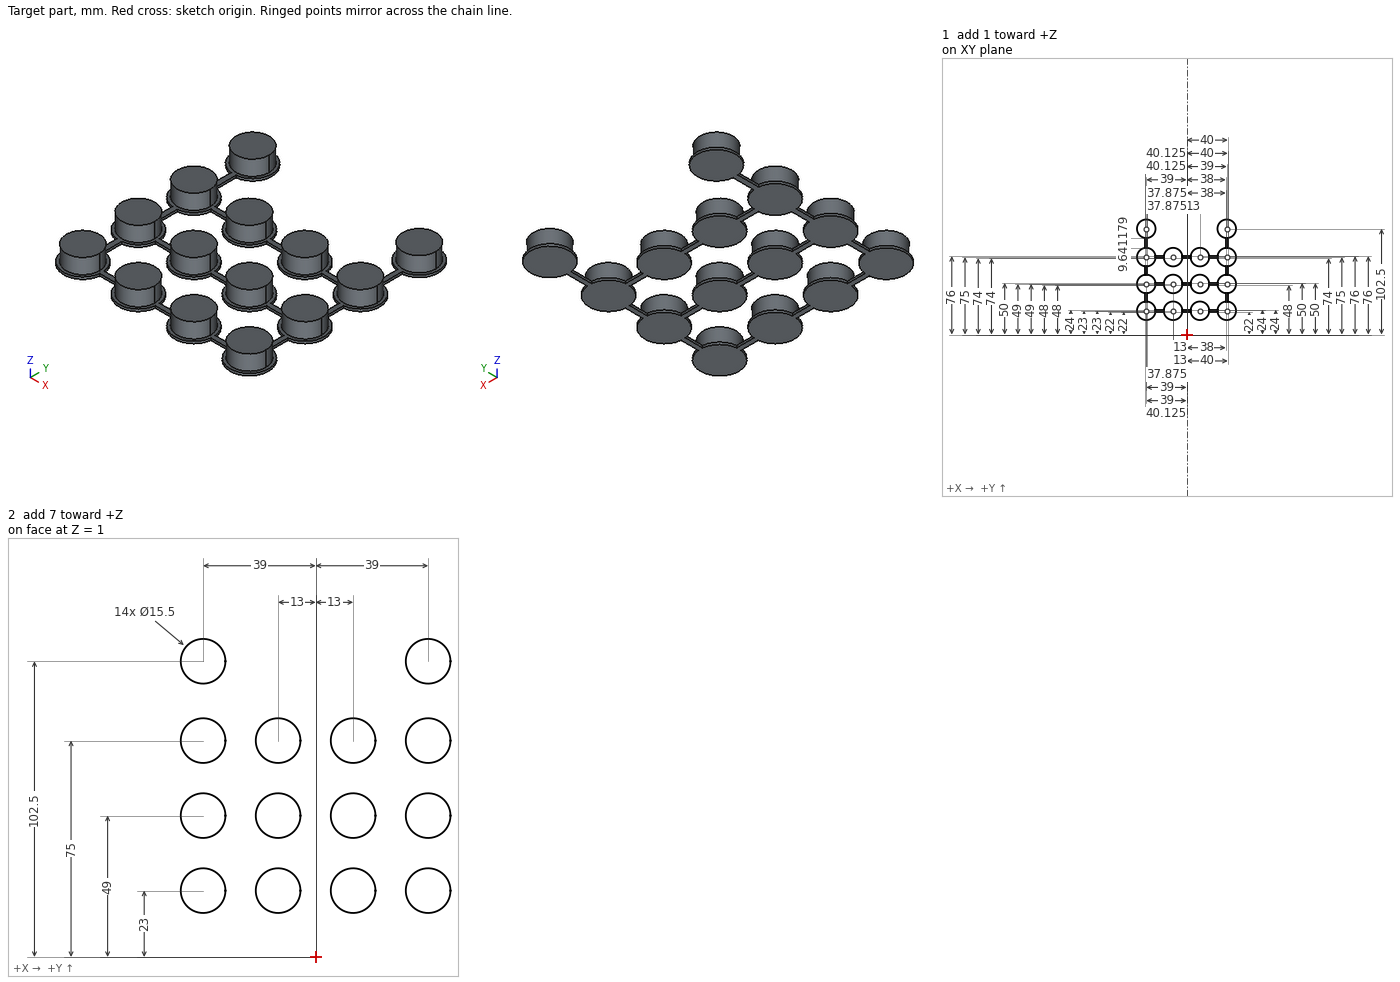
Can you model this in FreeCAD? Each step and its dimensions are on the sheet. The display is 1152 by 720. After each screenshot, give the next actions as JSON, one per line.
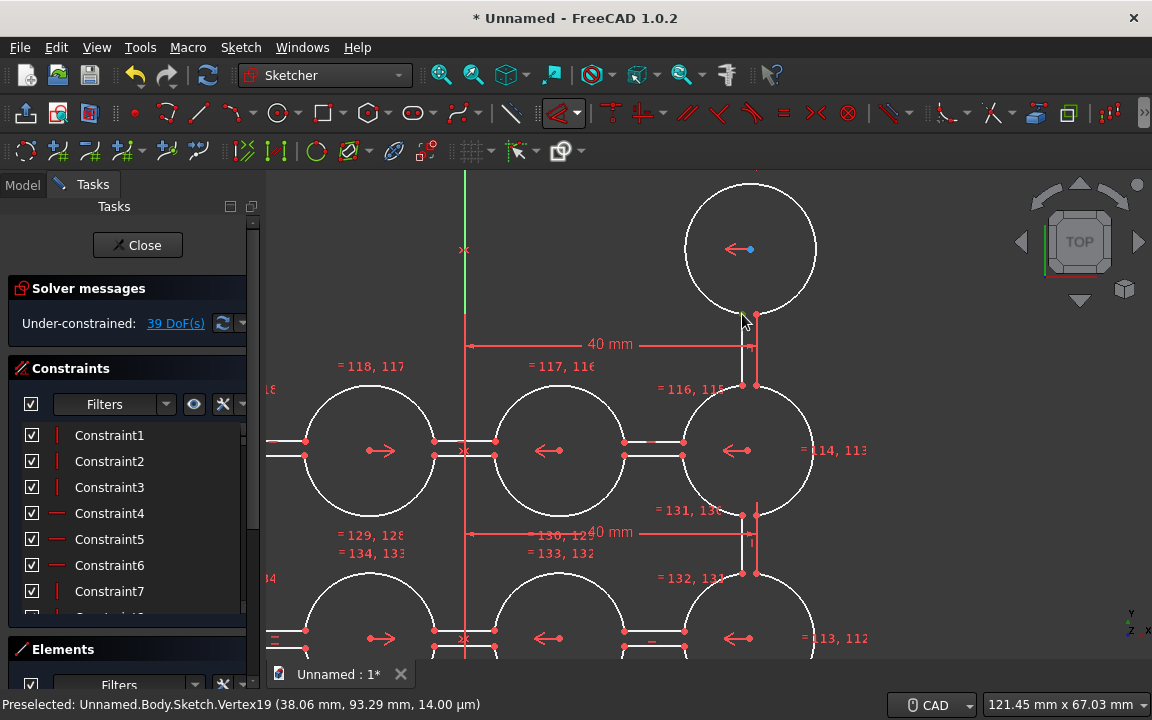
{"action": "left_click", "coordinate": [580, 114]}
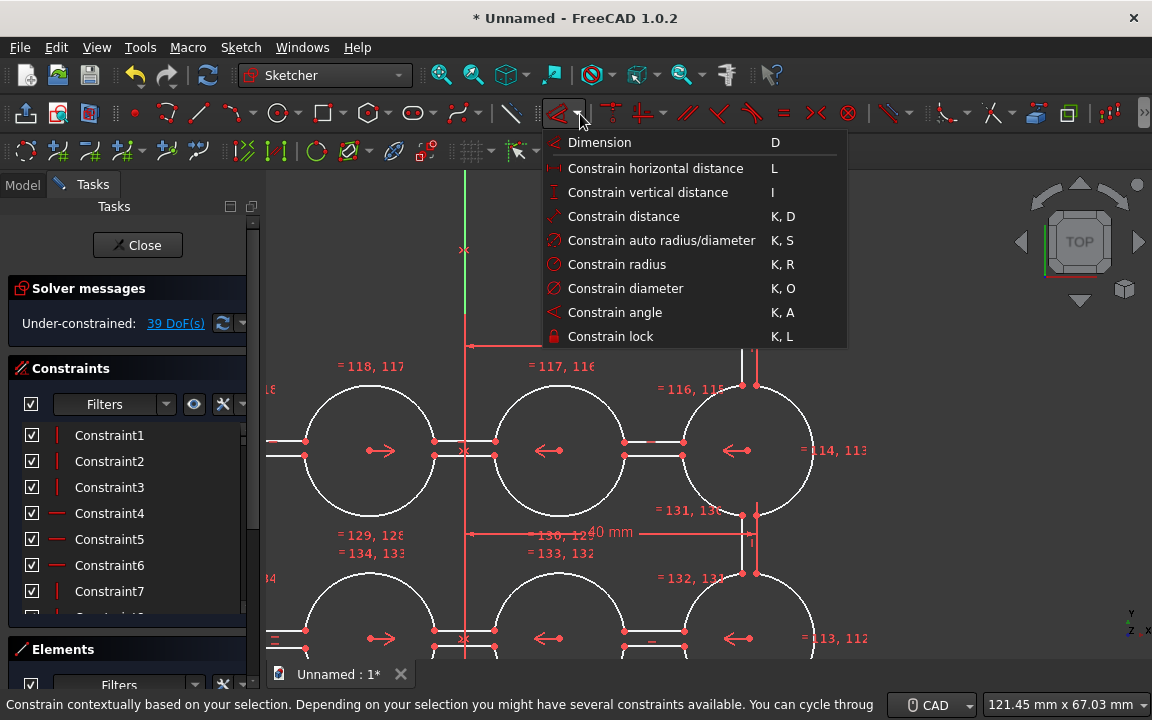
{"action": "left_click", "coordinate": [695, 168]}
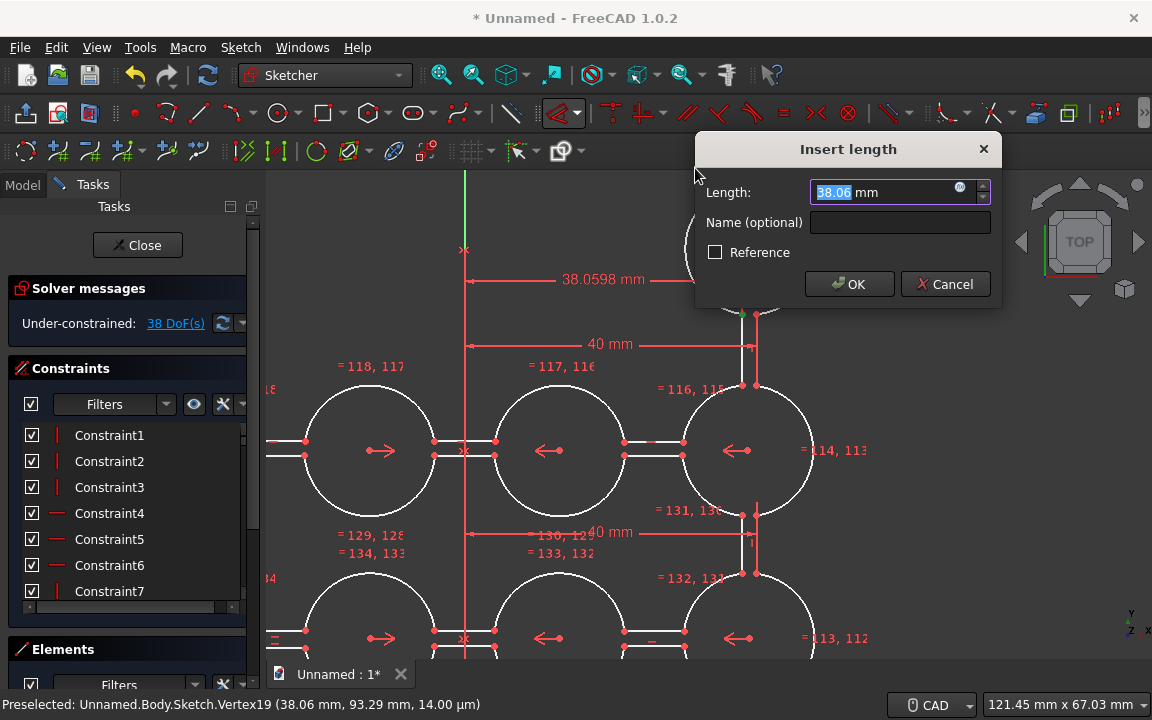
{"action": "type", "text": "38"}
{"action": "key", "text": "Return"}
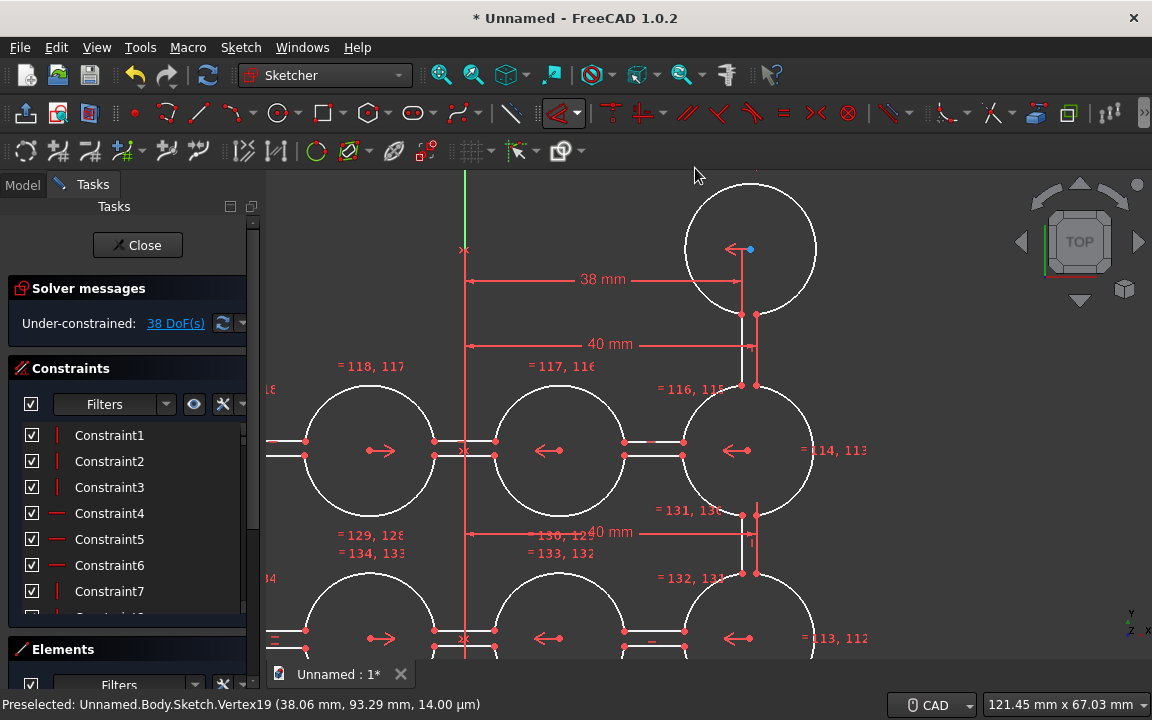
{"action": "left_click", "coordinate": [683, 442]}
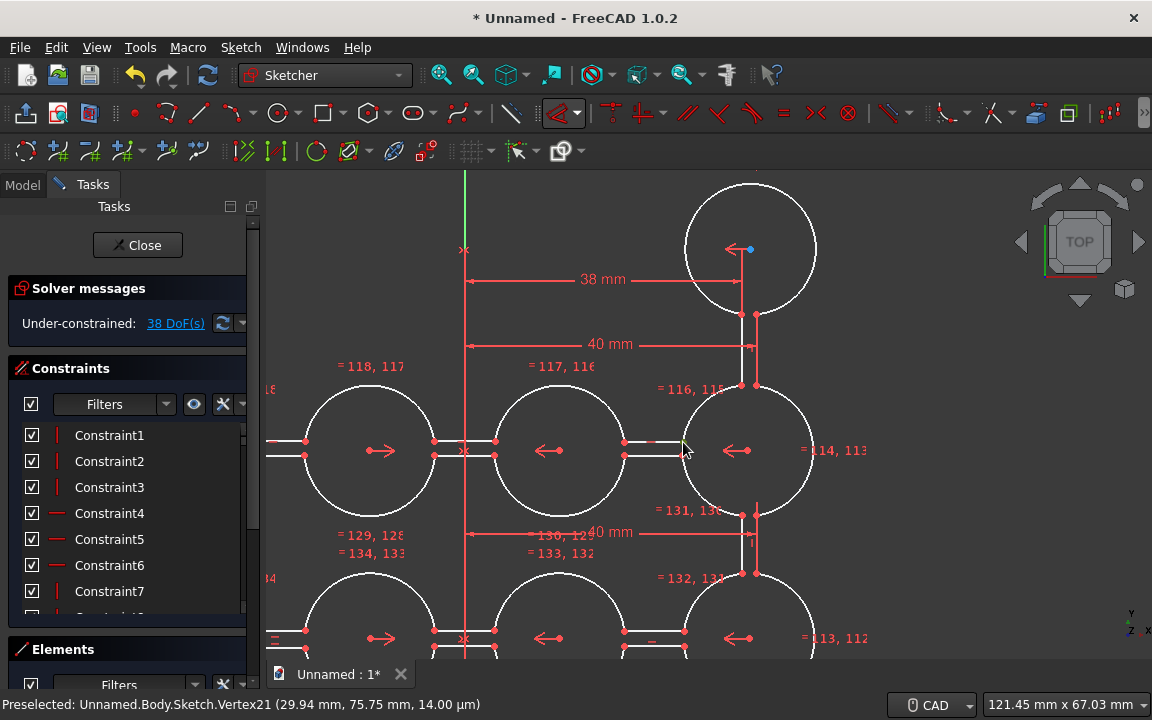
{"action": "left_click", "coordinate": [580, 114]}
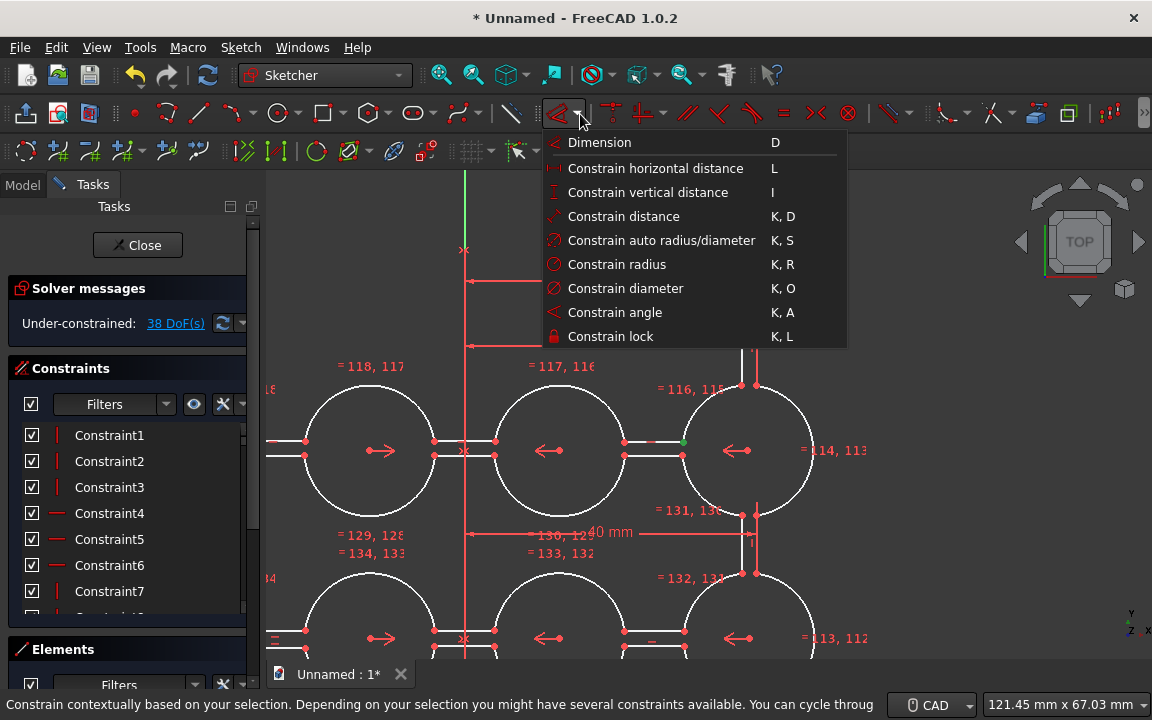
{"action": "left_click", "coordinate": [695, 192]}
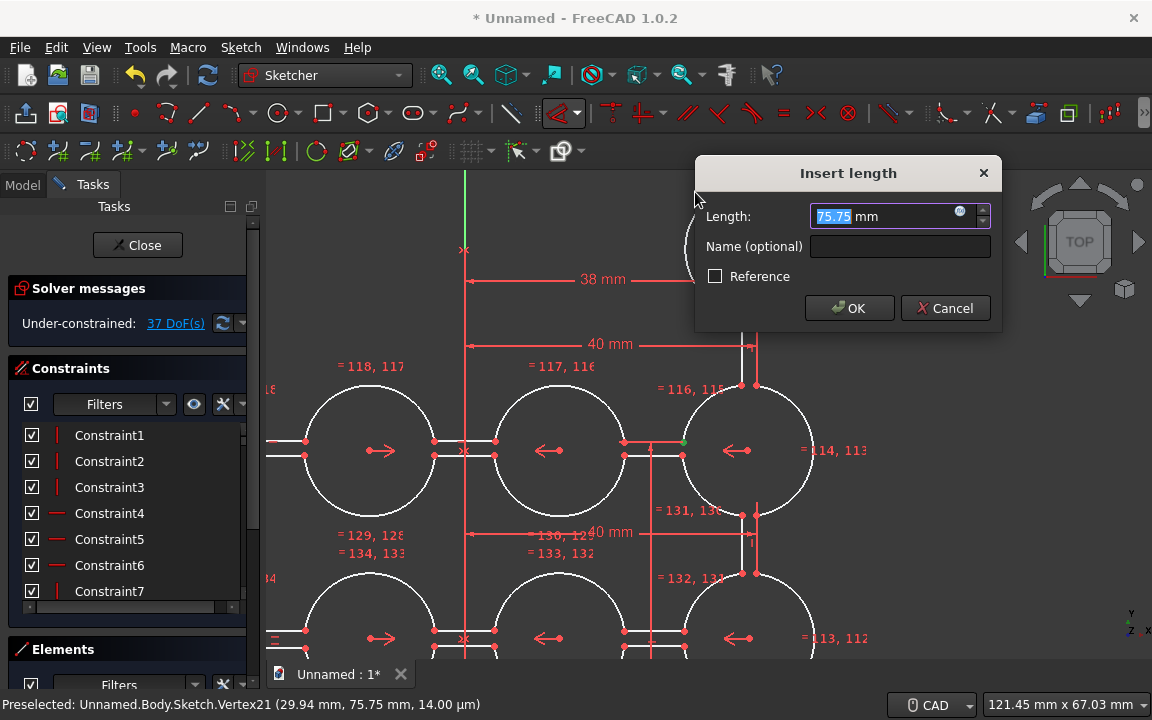
{"action": "type", "text": "76"}
{"action": "key", "text": "Return"}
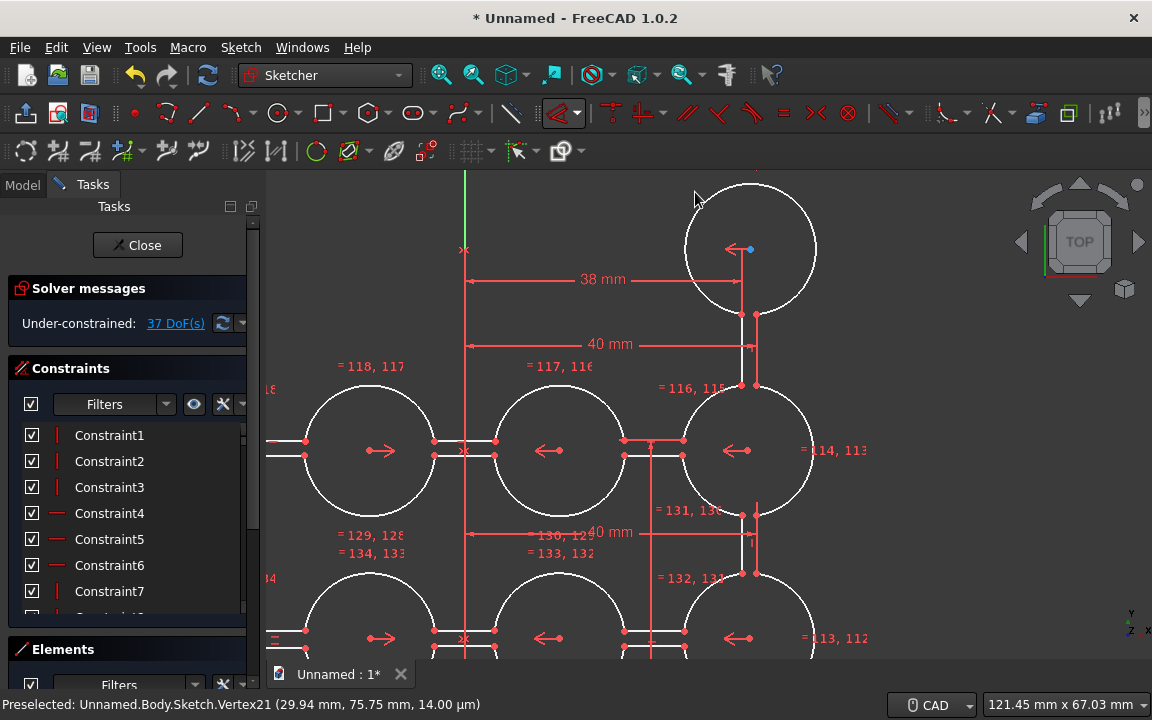
{"action": "left_click", "coordinate": [495, 441]}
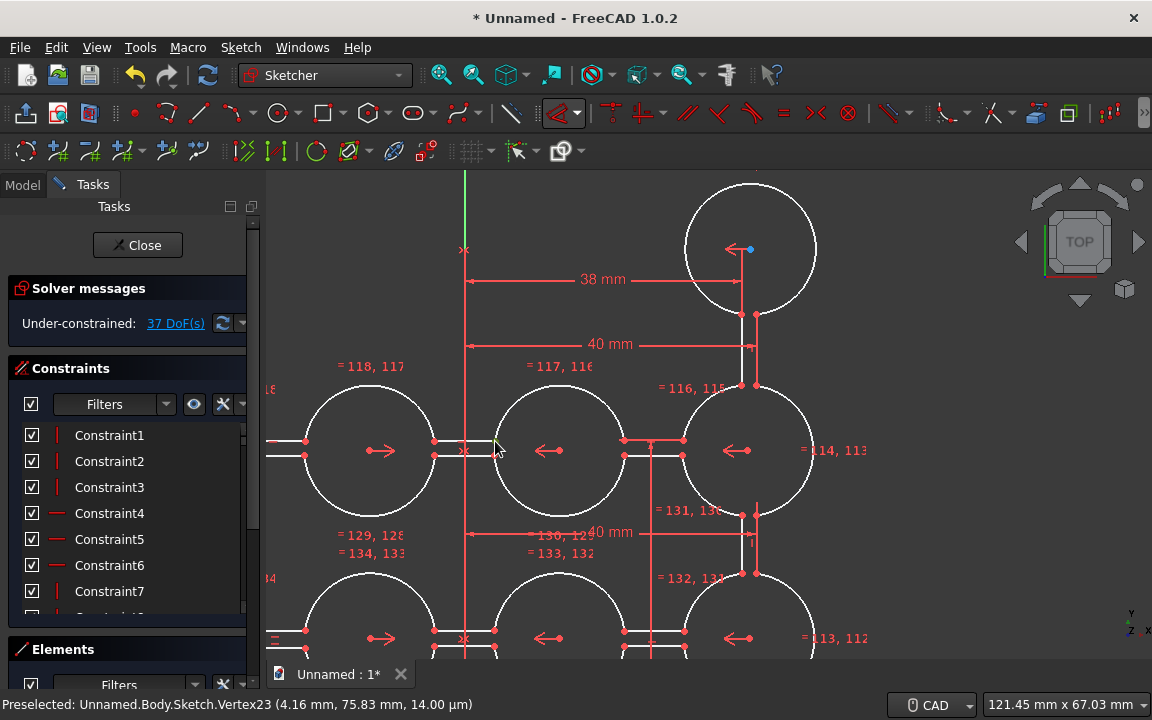
{"action": "left_click", "coordinate": [580, 114]}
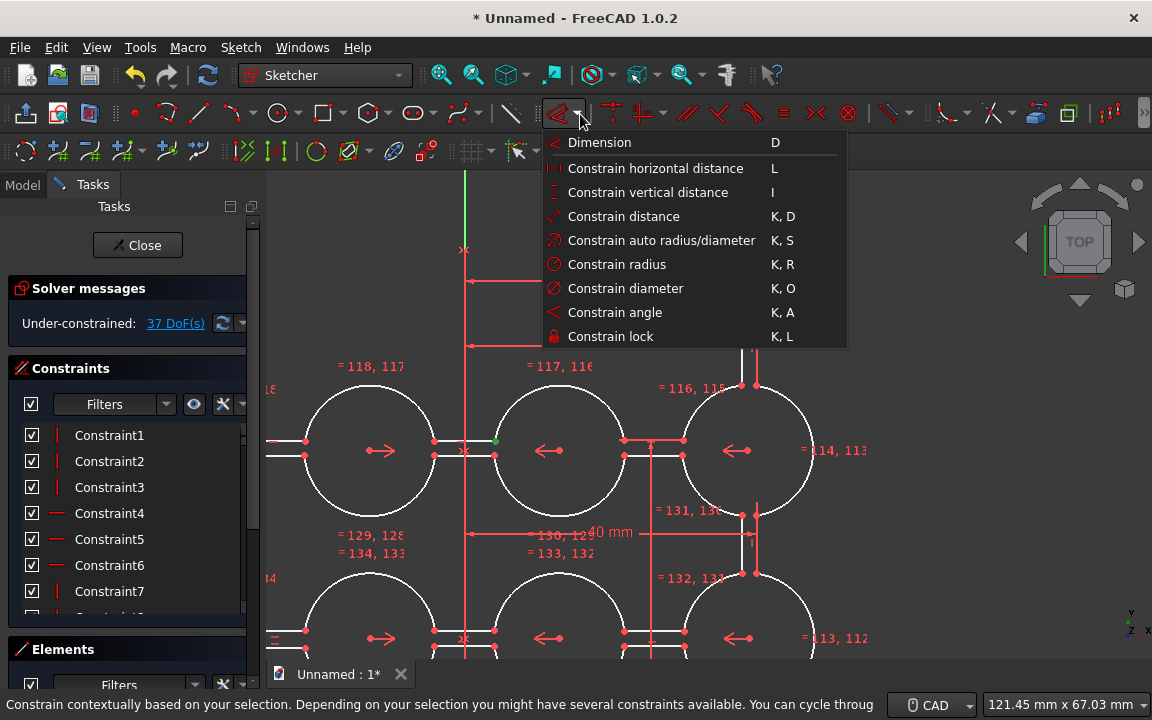
{"action": "left_click", "coordinate": [695, 192]}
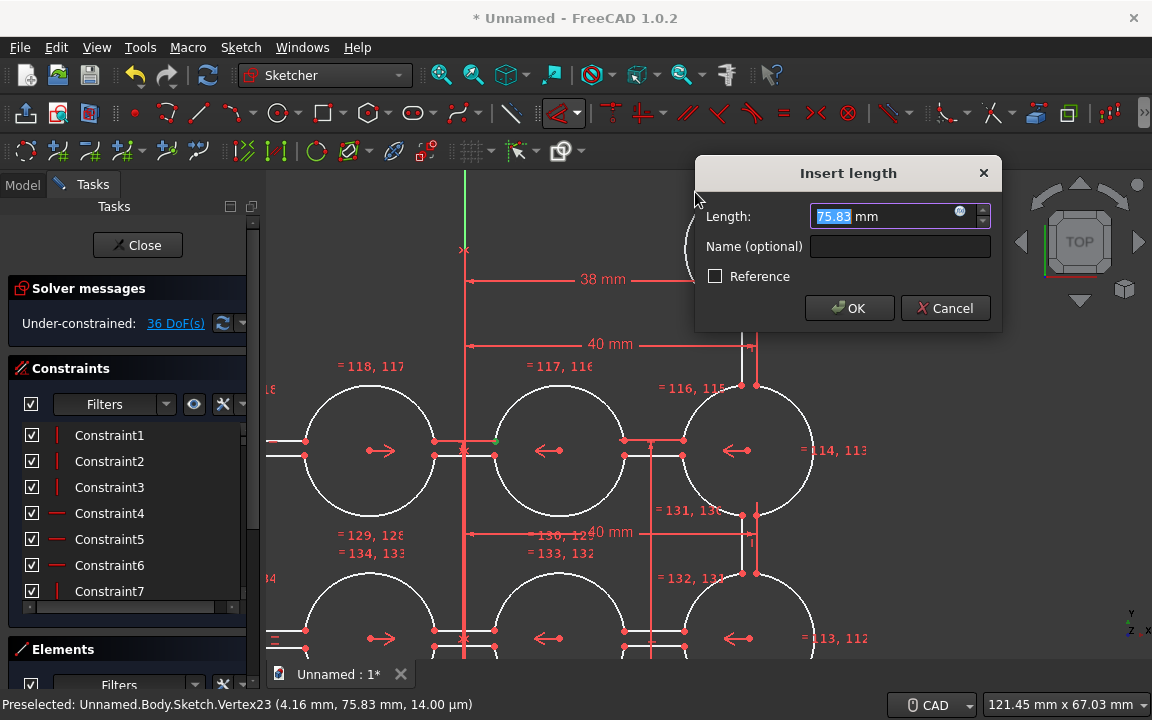
{"action": "type", "text": "76"}
{"action": "key", "text": "Return"}